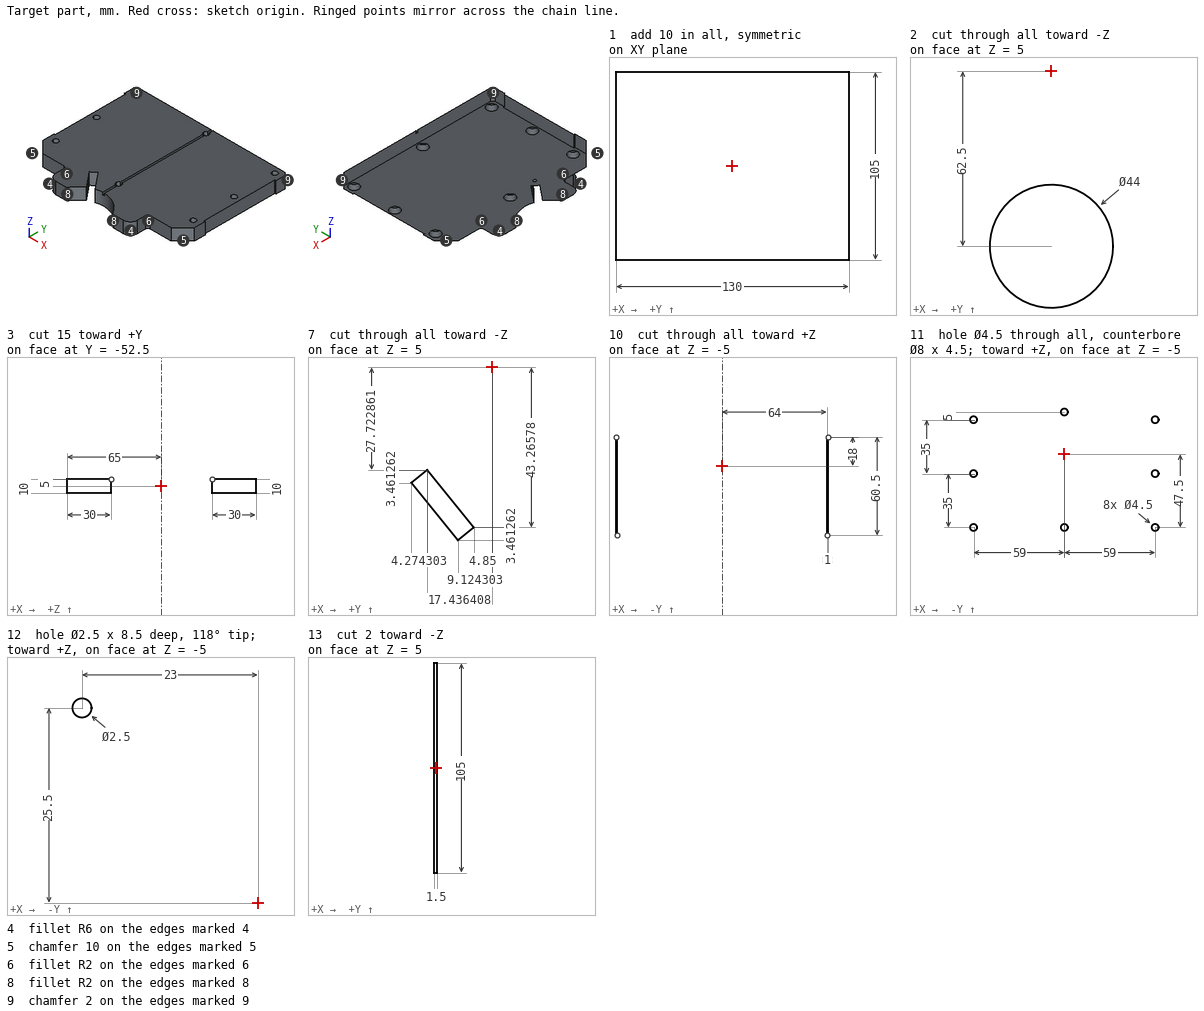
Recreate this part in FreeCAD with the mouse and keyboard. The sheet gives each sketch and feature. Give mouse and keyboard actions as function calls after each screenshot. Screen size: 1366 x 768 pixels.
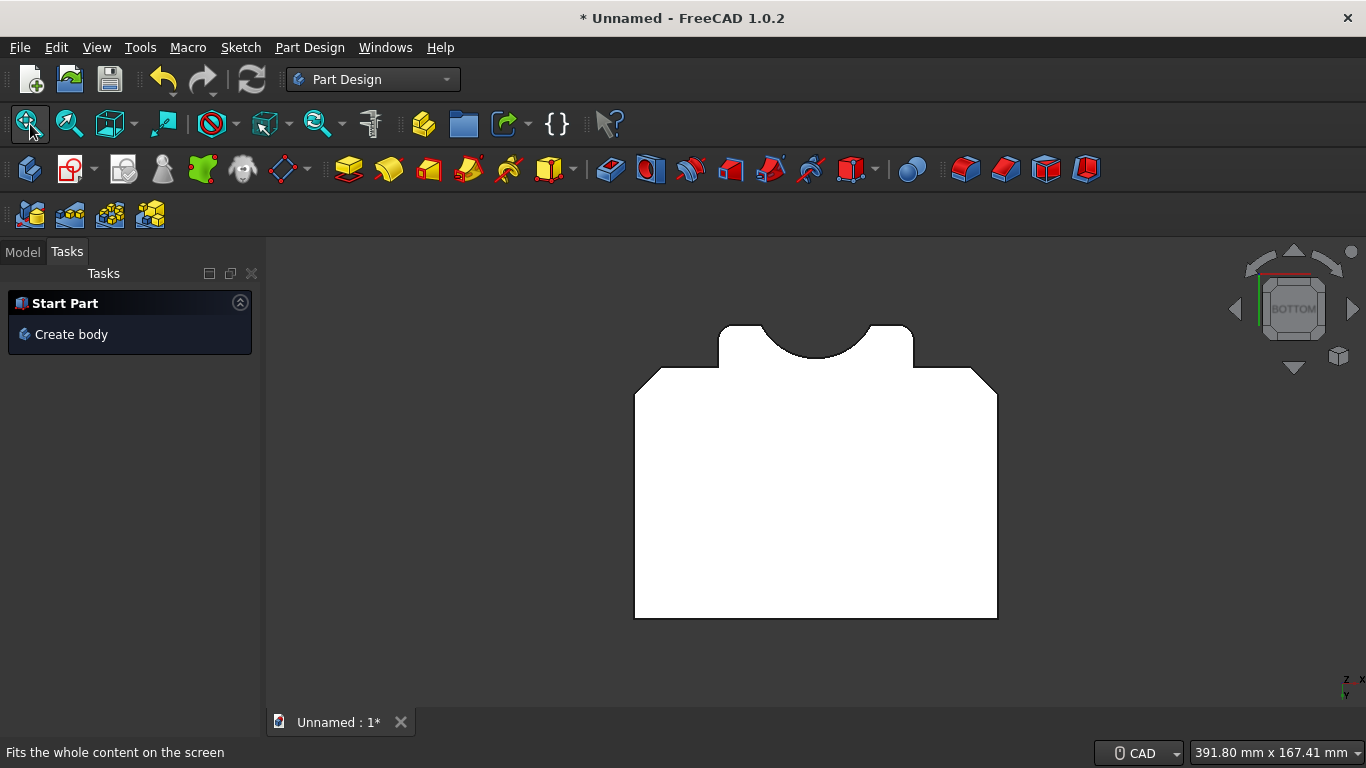
key(4)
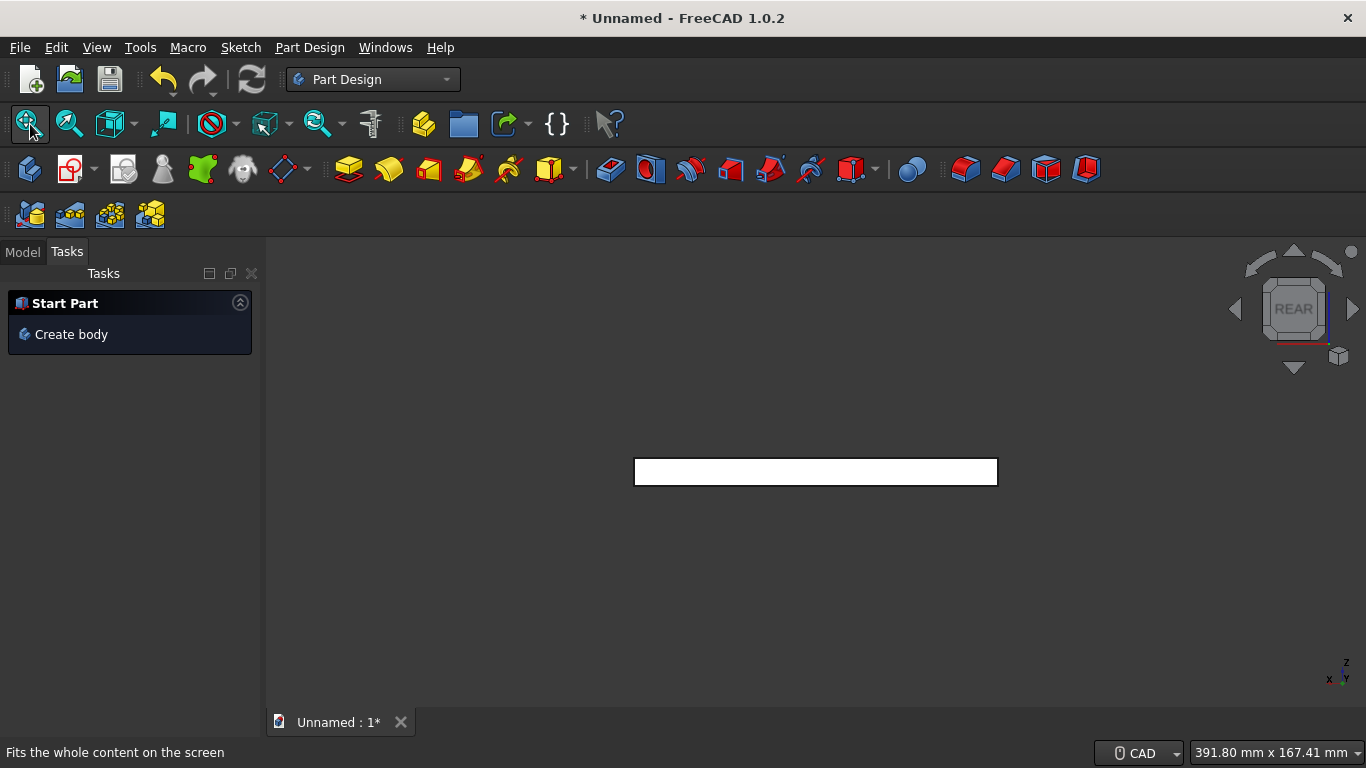
click(30, 124)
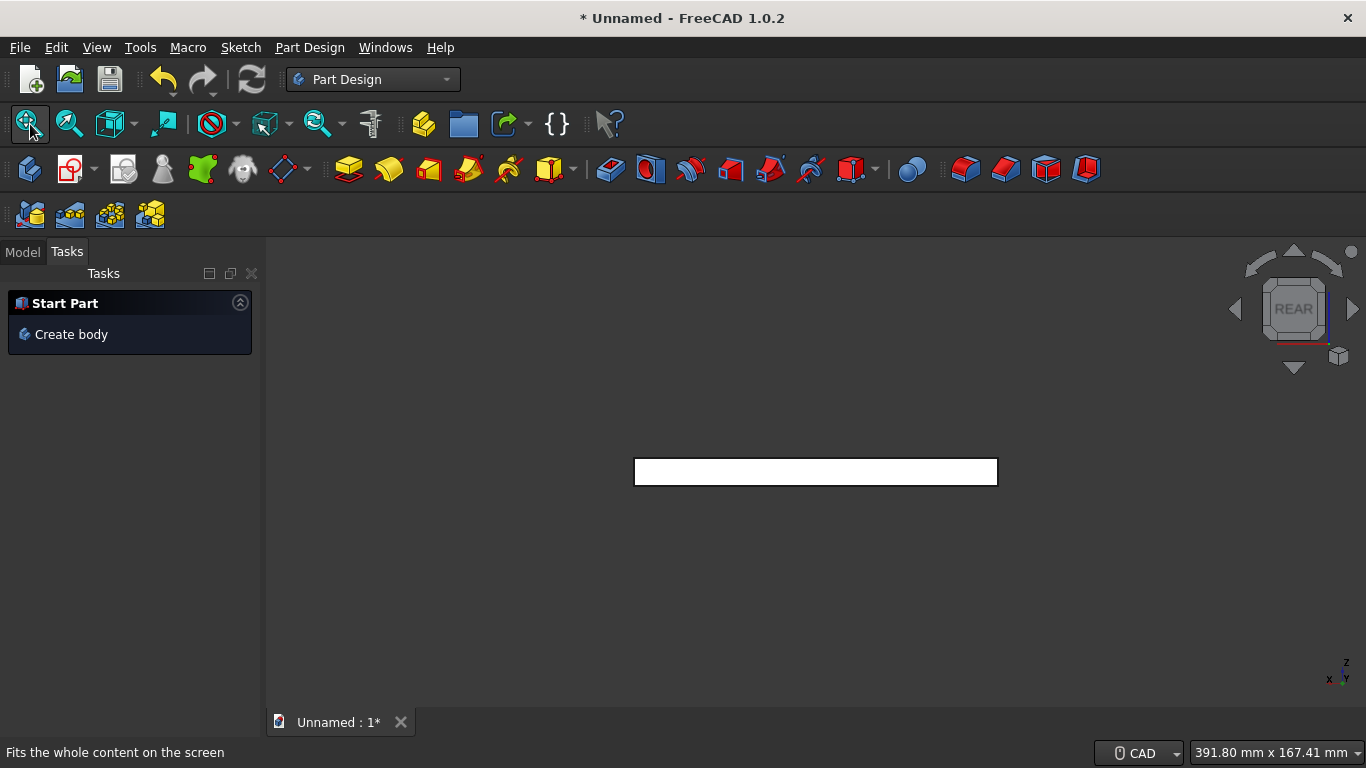
key(6)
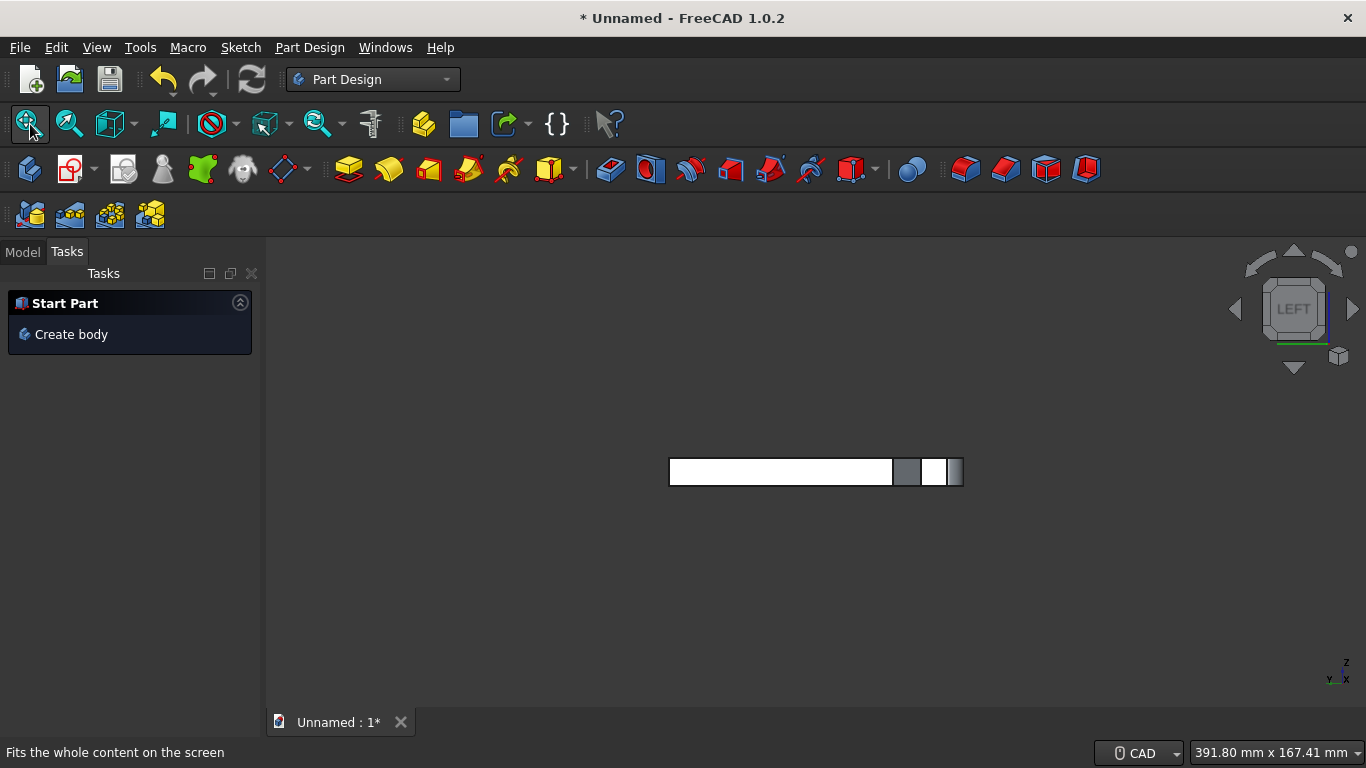
click(30, 124)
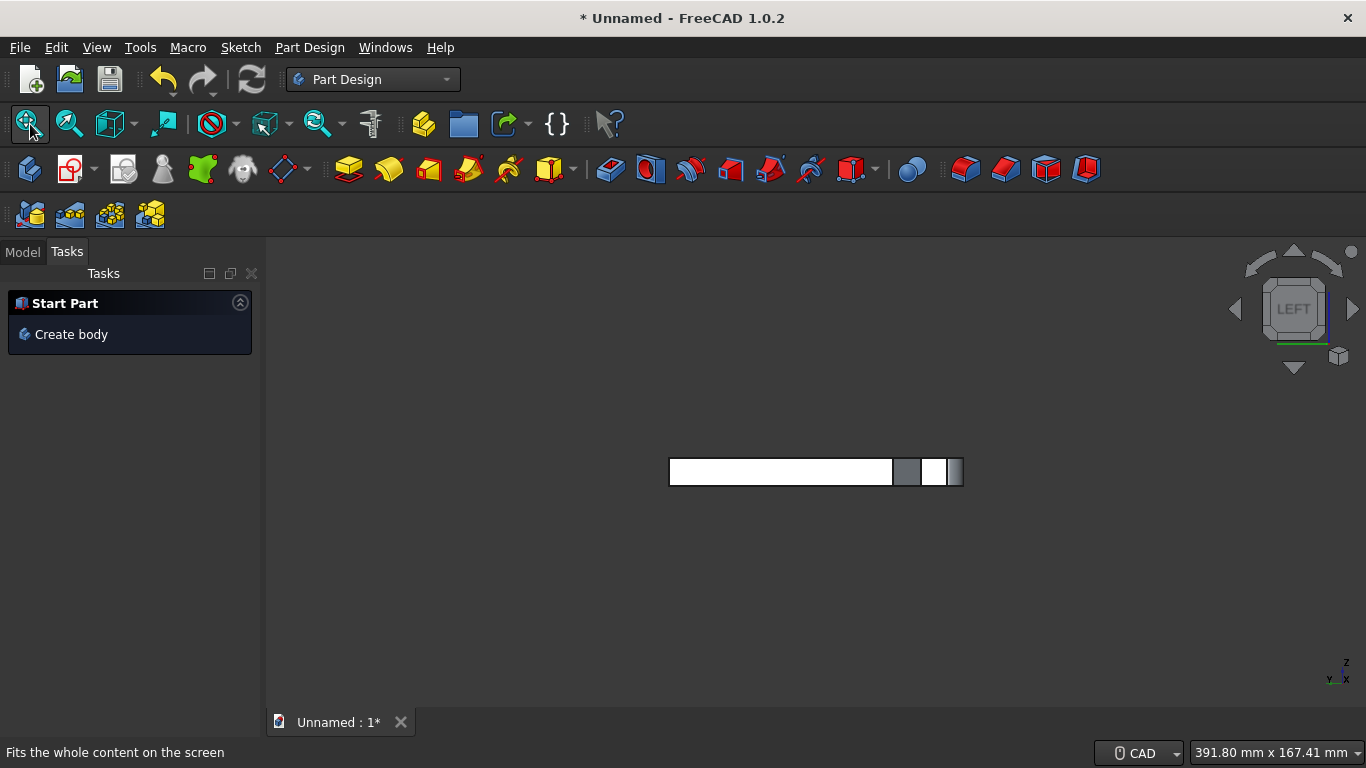
key(v)
key(3)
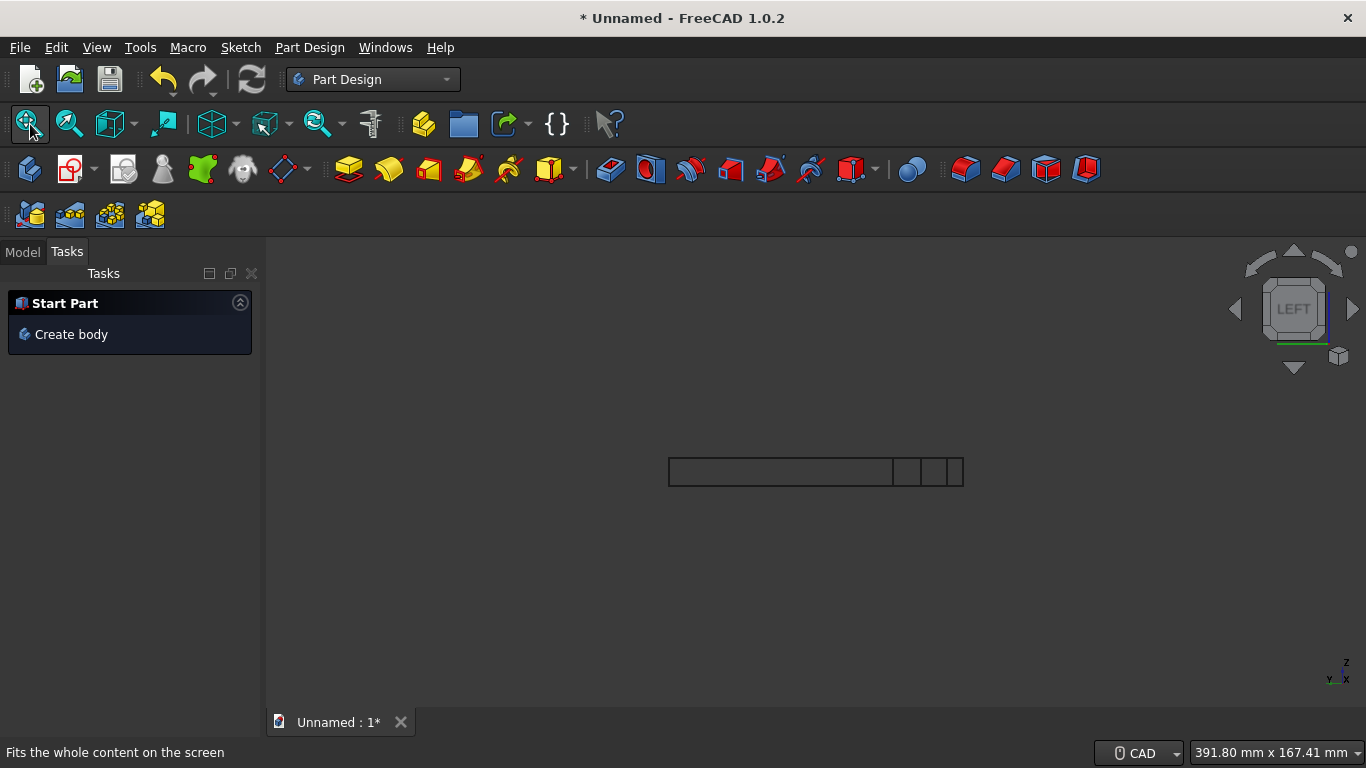
key(0)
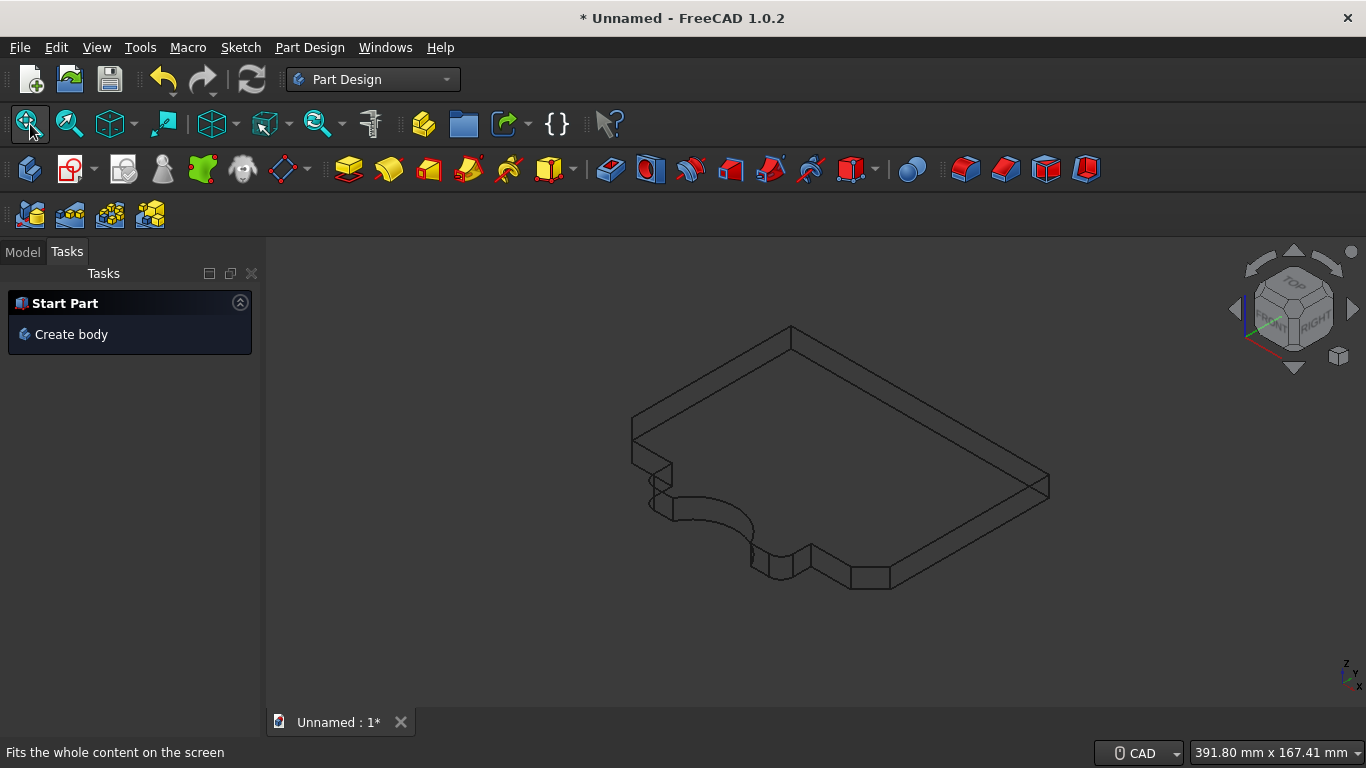
click(672, 474)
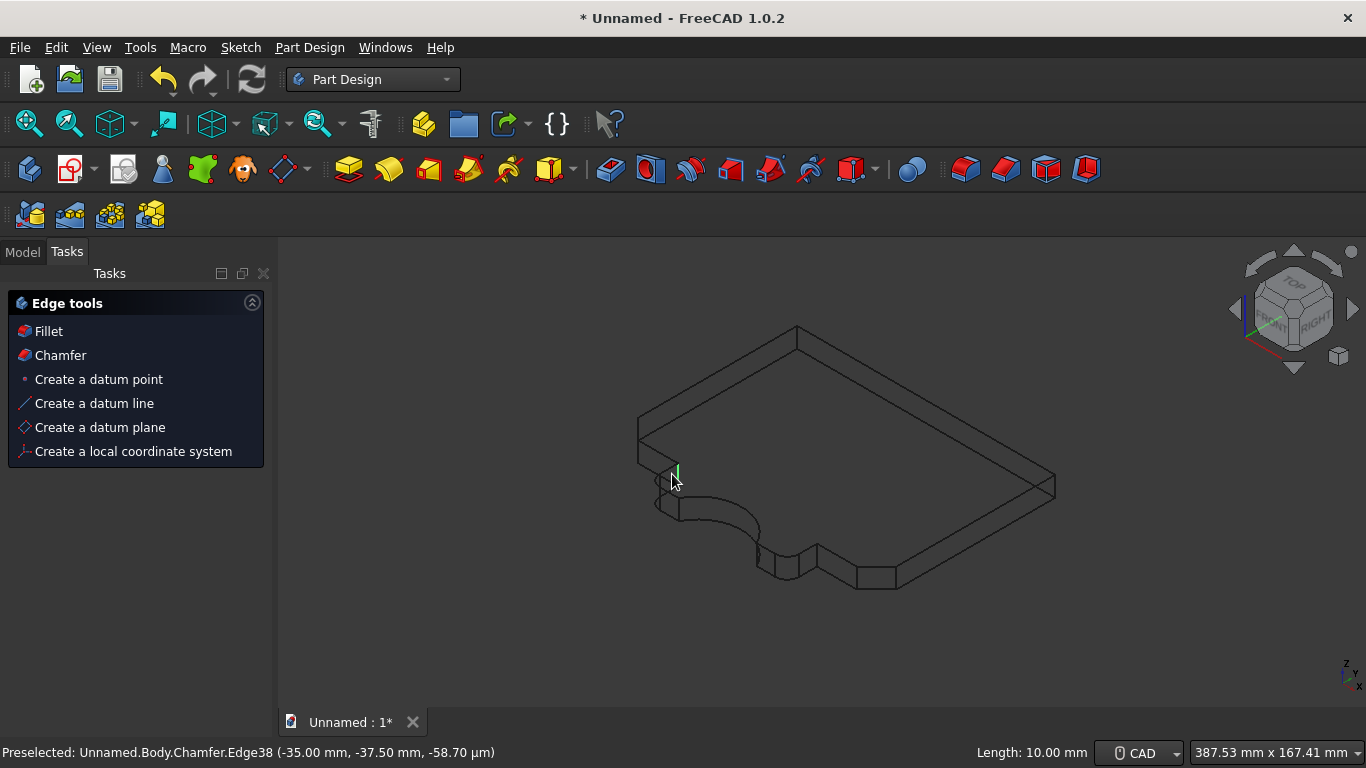
click(817, 554, ctrl)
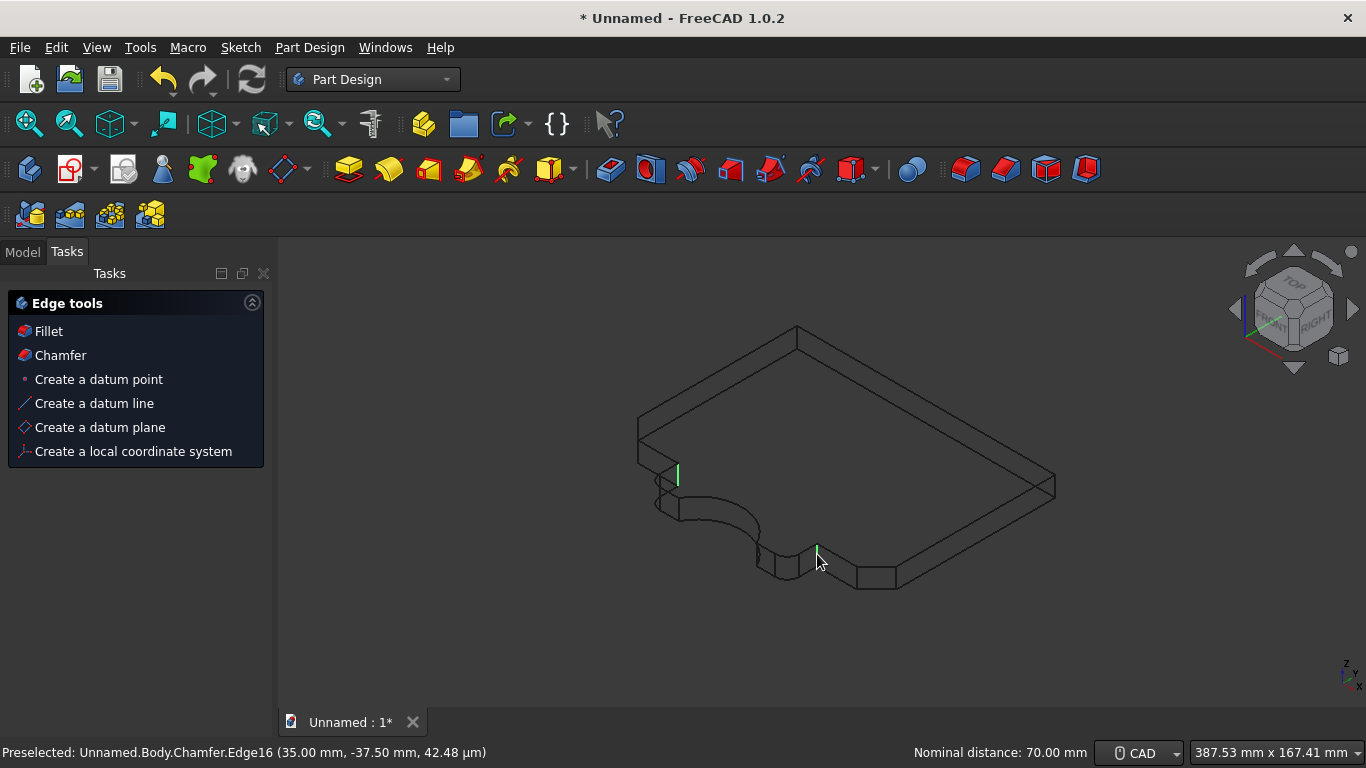
key(v)
key(1)